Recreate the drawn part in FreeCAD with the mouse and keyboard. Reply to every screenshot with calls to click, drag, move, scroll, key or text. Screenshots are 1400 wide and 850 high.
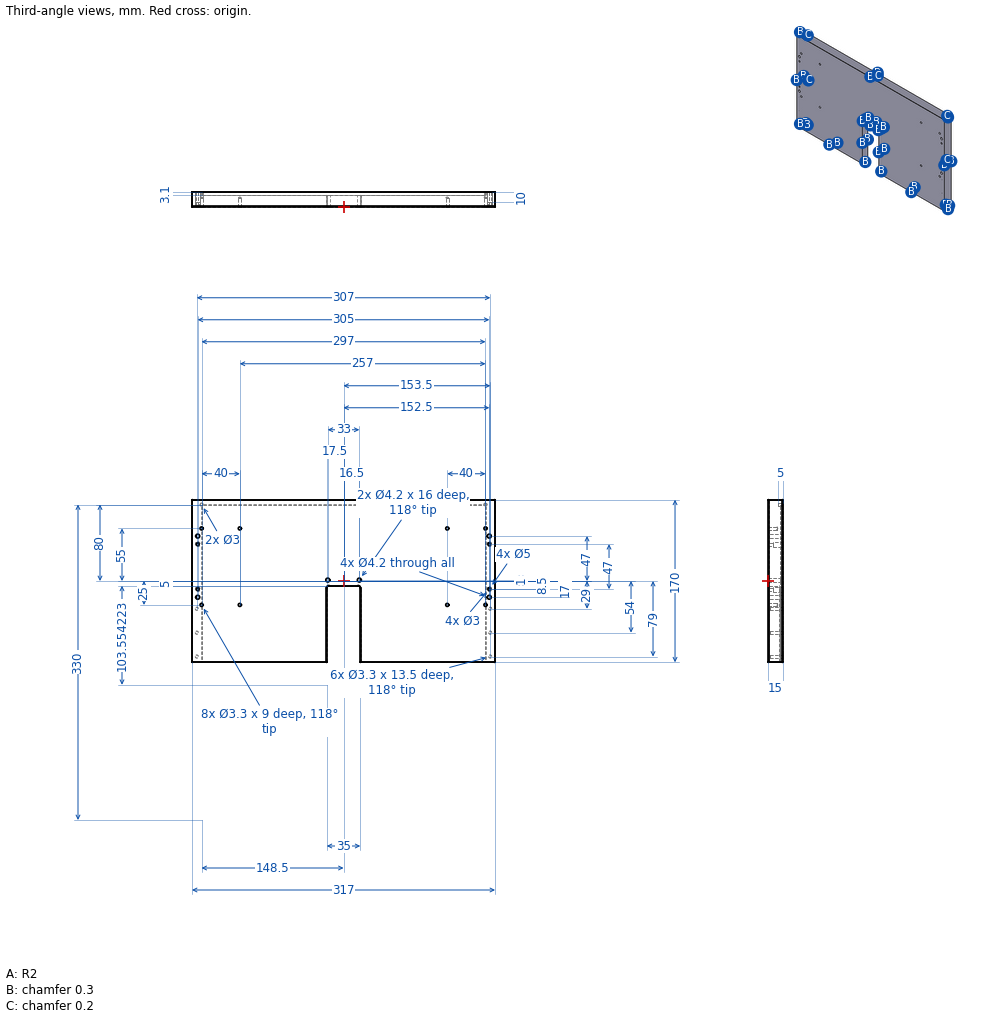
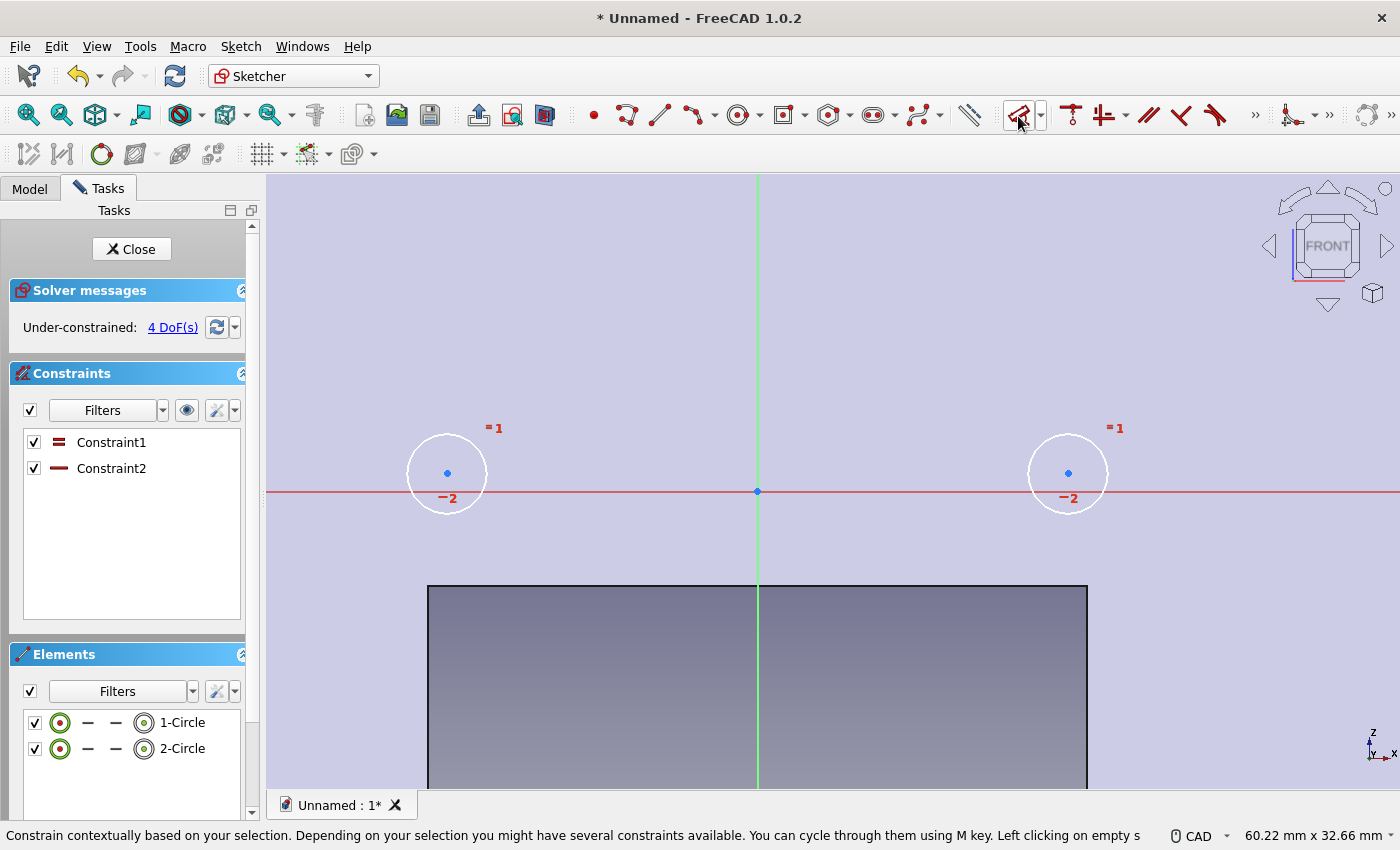
click(1096, 446)
click(1119, 423)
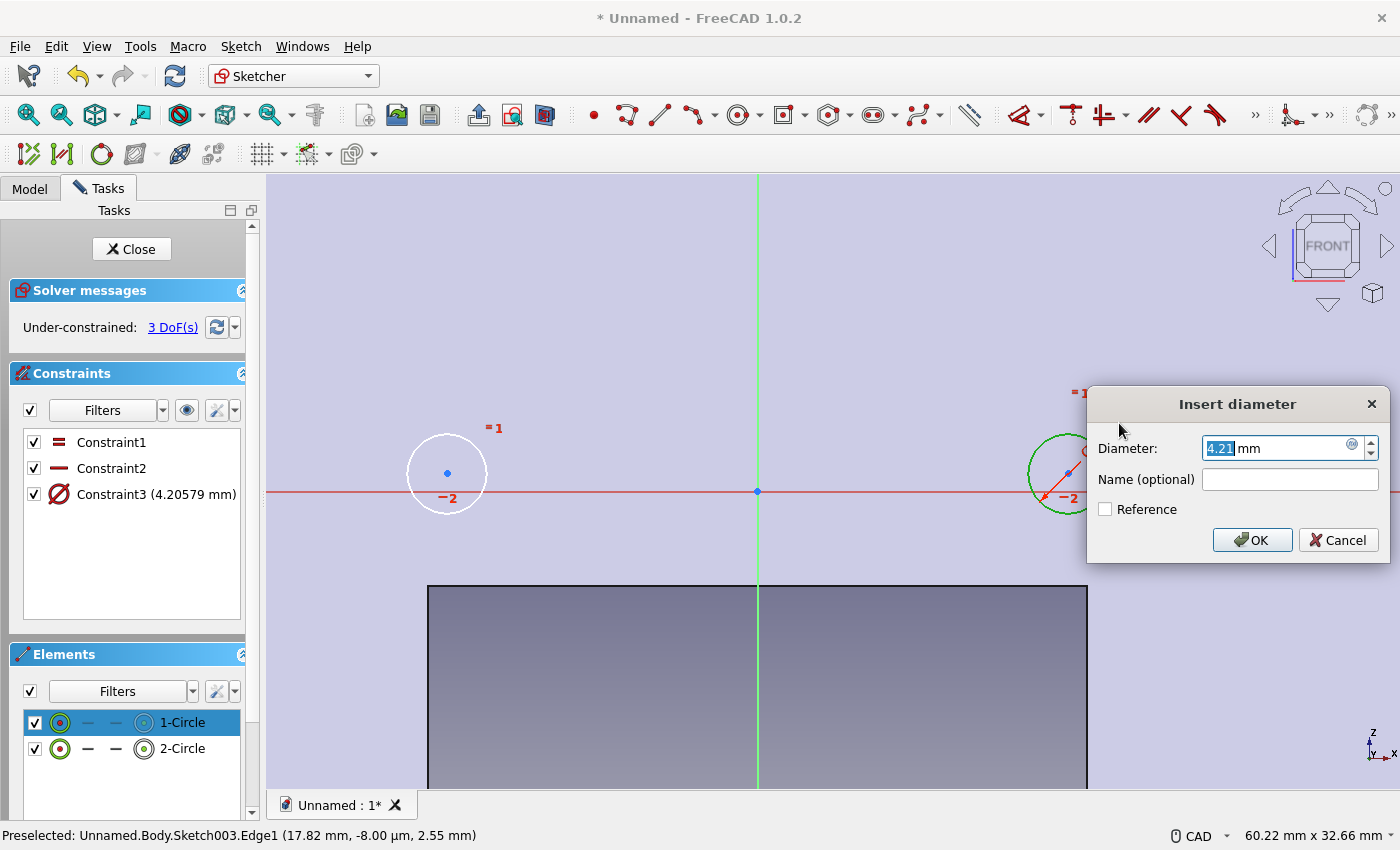
text(4.2)
key(Return)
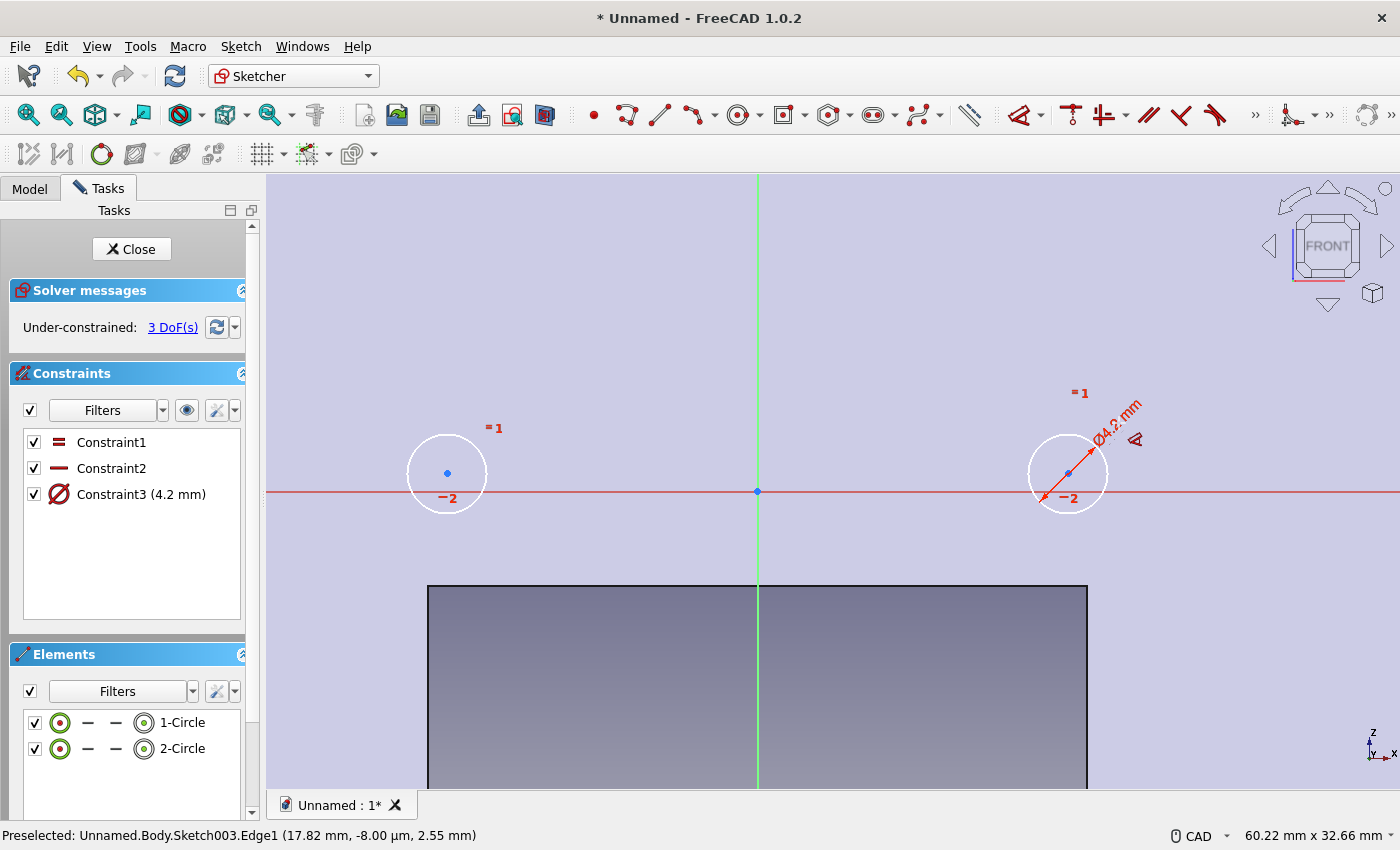
scroll(1068, 474, up, 4)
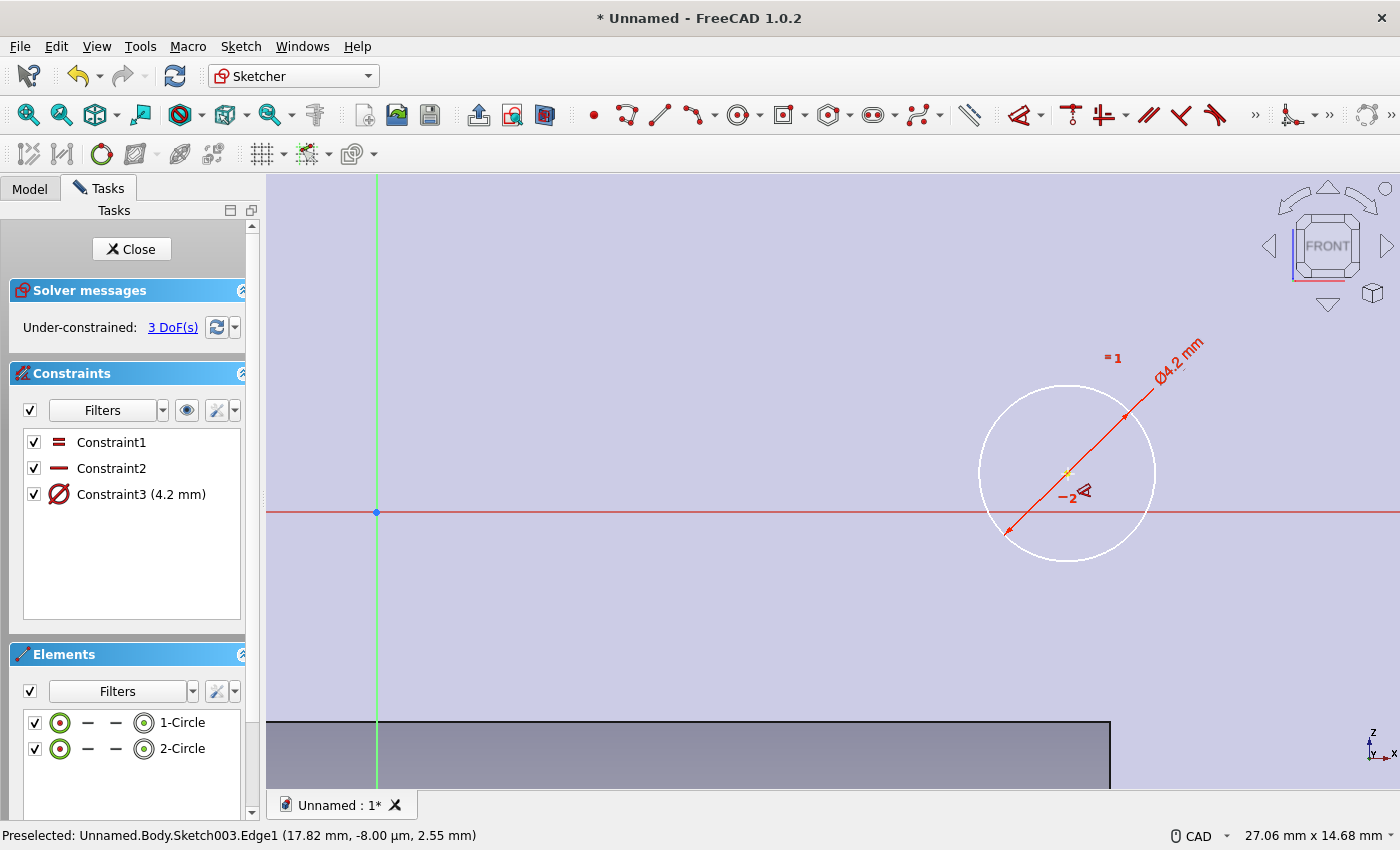
click(1067, 473)
click(1101, 493)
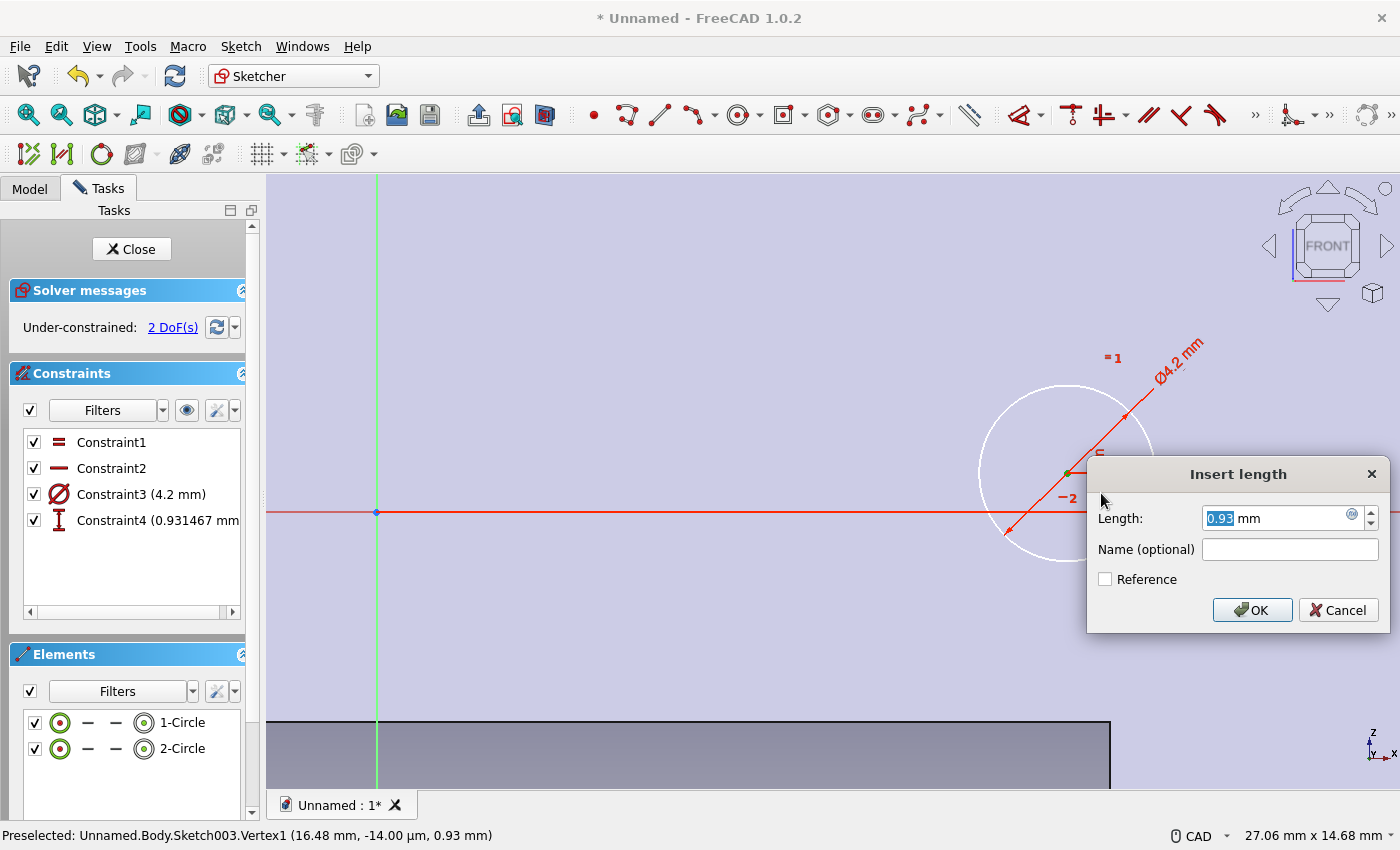
text(1)
key(Return)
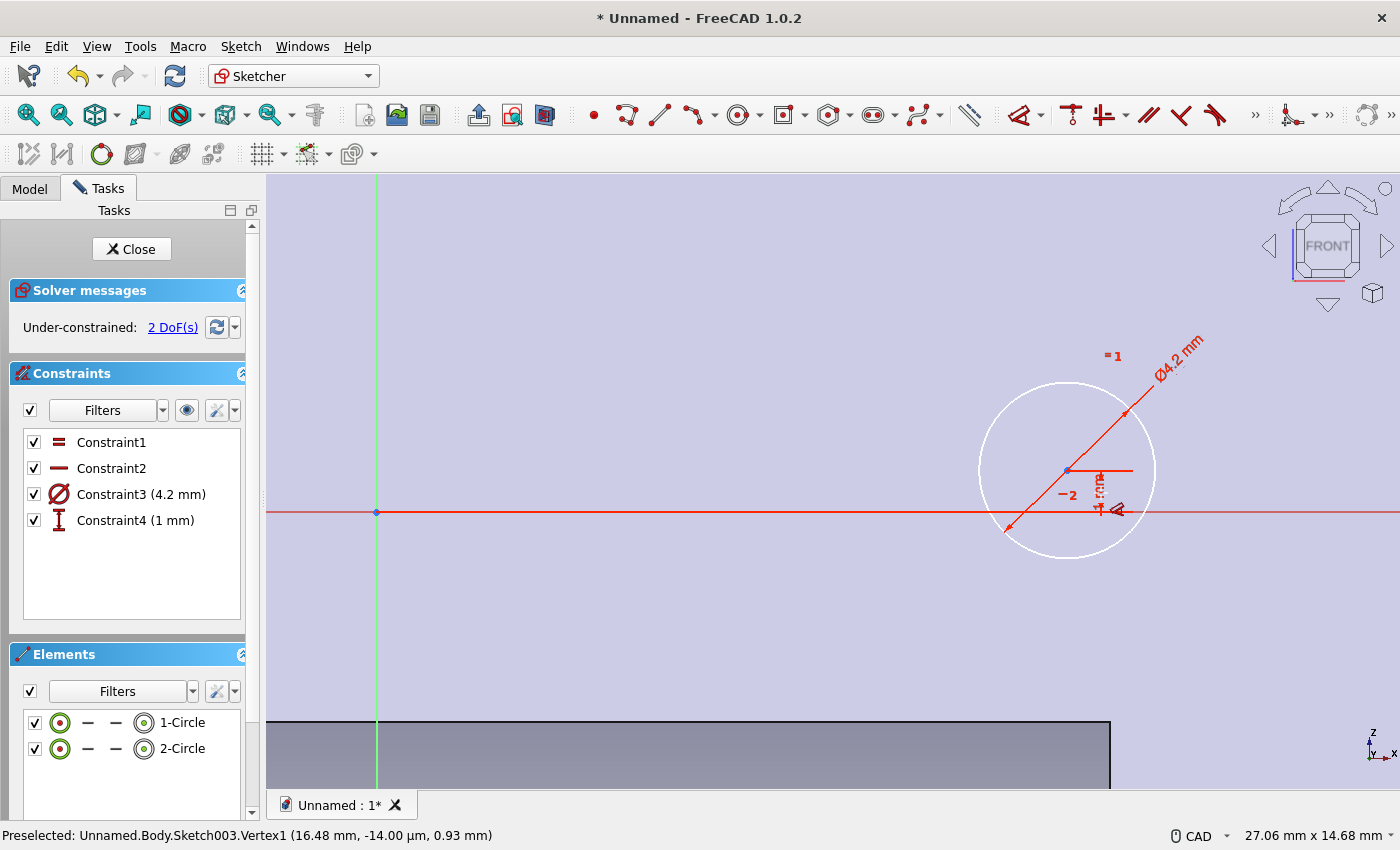
click(1067, 471)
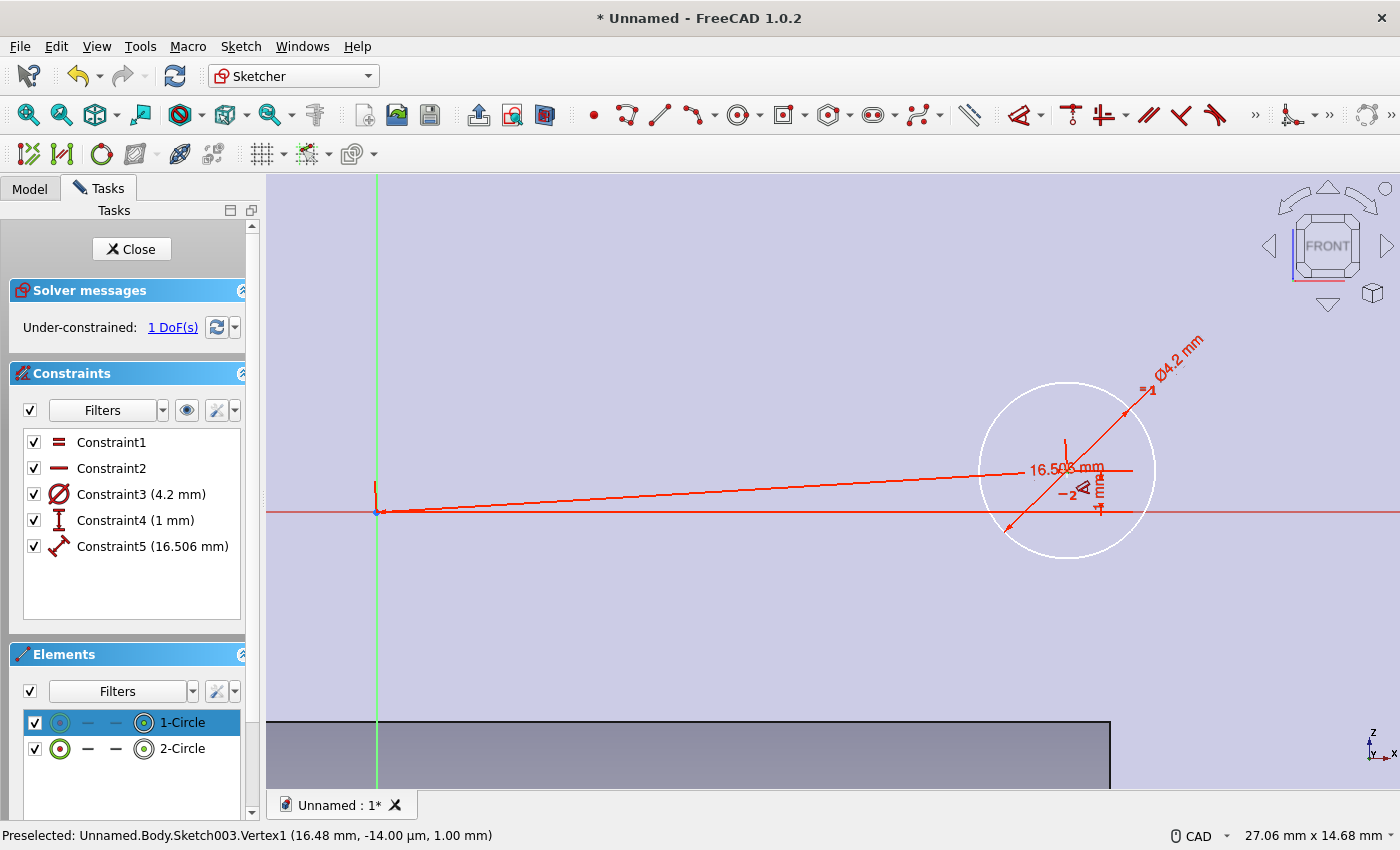
scroll(1081, 490, down, 4)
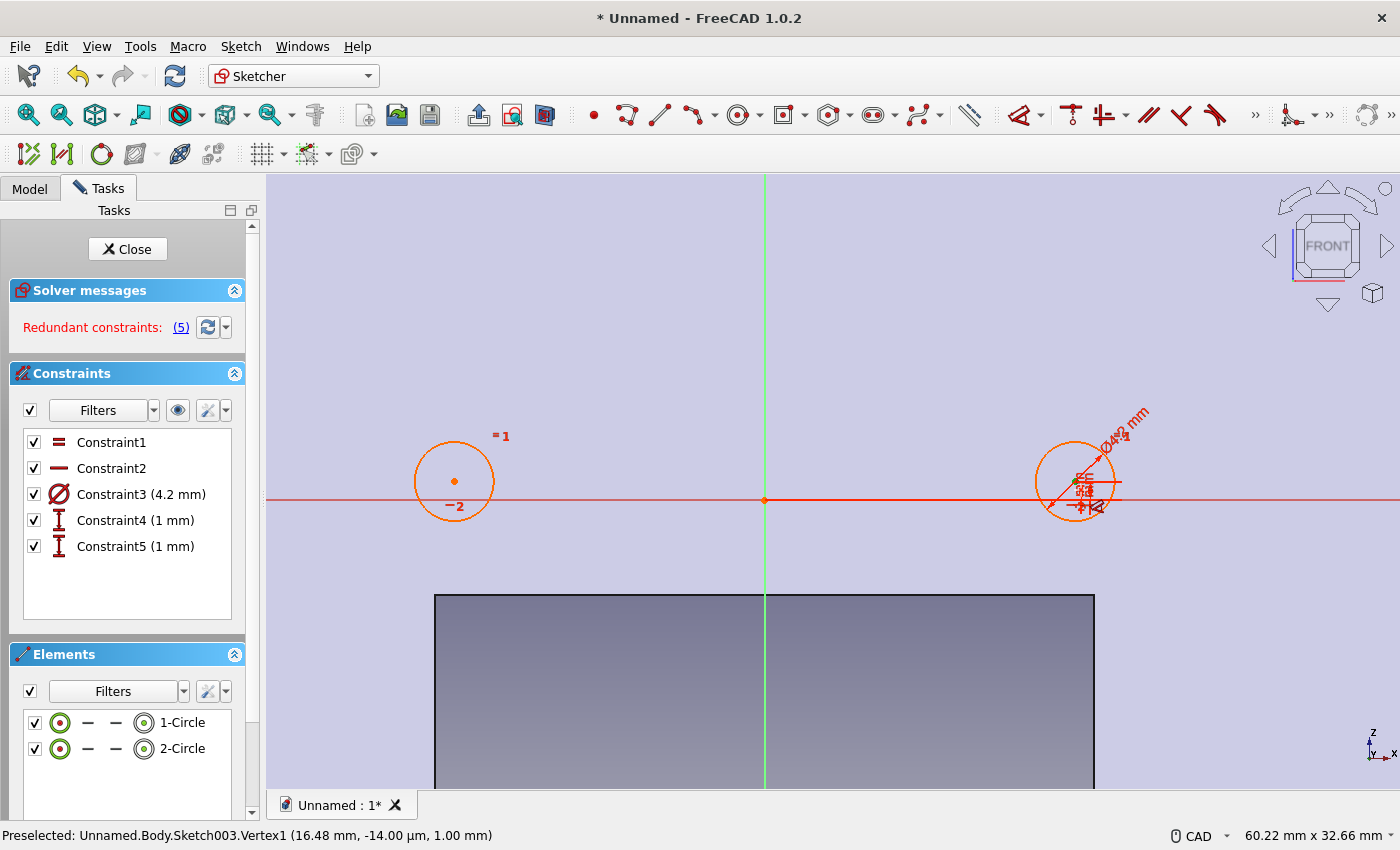
click(454, 482)
click(622, 516)